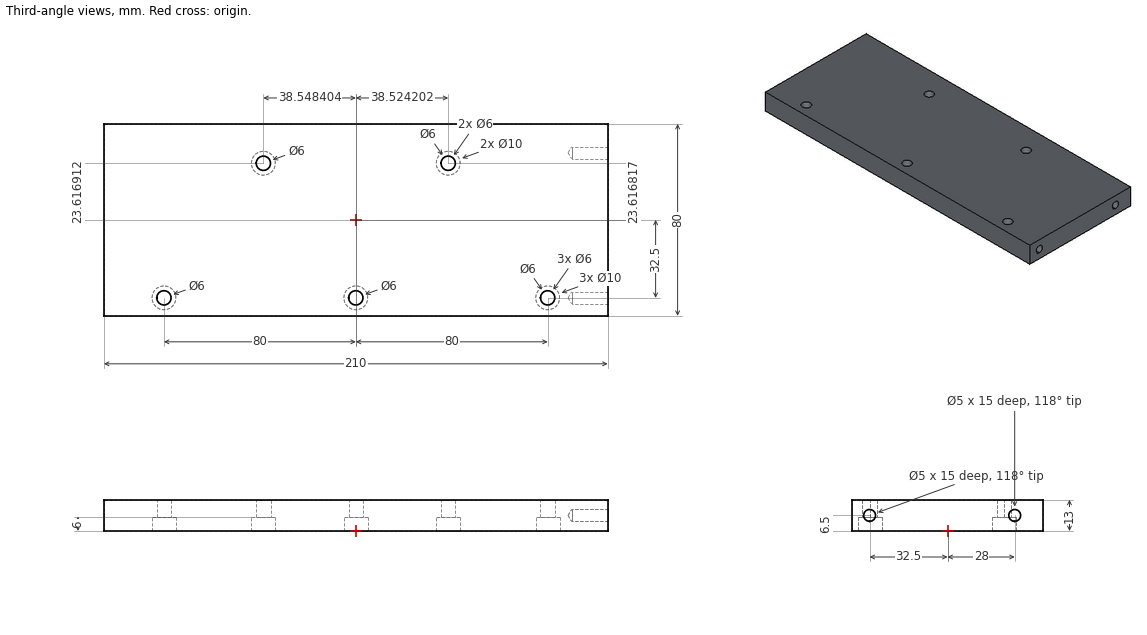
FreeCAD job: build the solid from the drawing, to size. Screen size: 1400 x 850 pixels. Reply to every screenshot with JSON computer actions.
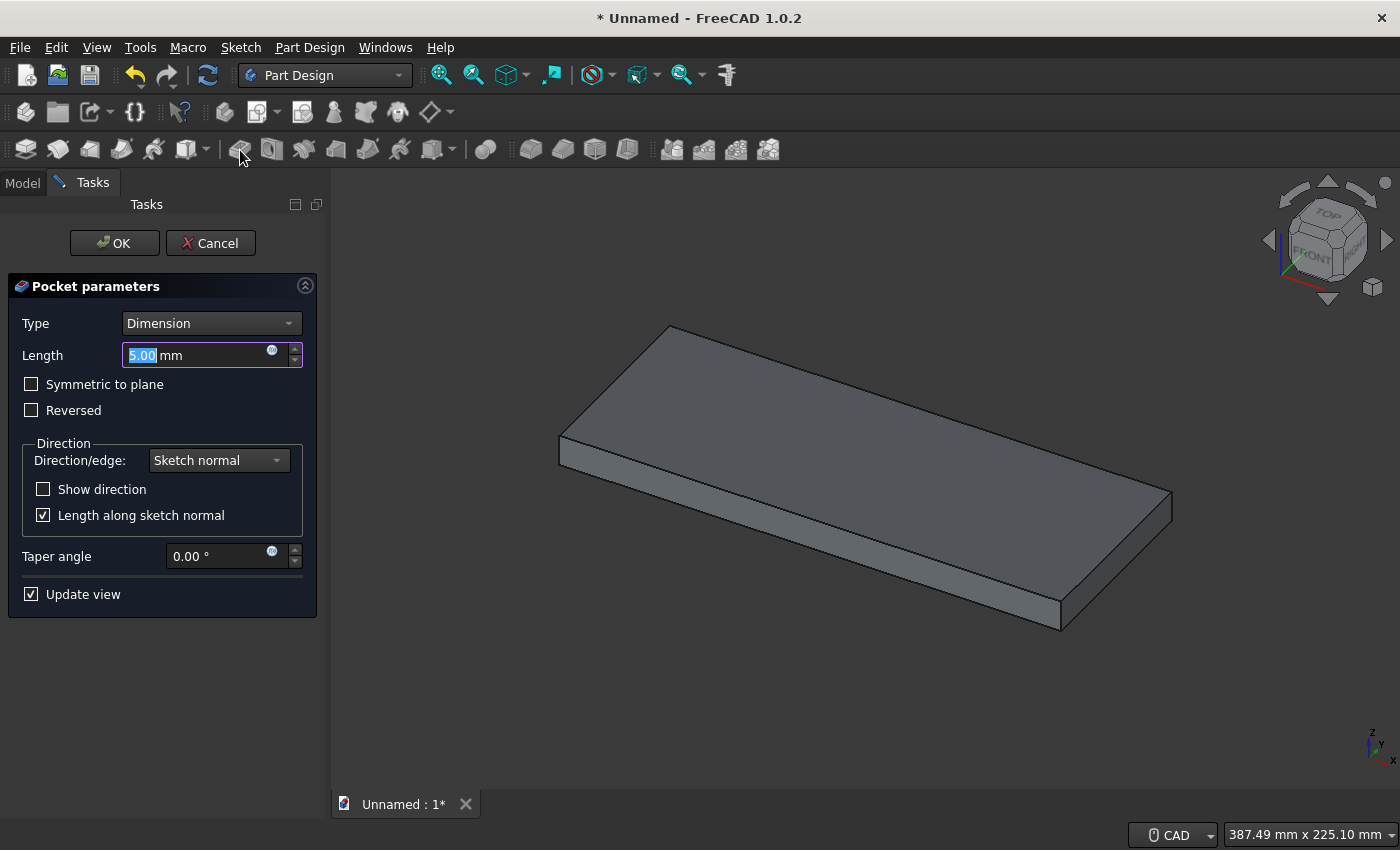
{"action": "type", "text": "6"}
{"action": "key", "text": "Tab"}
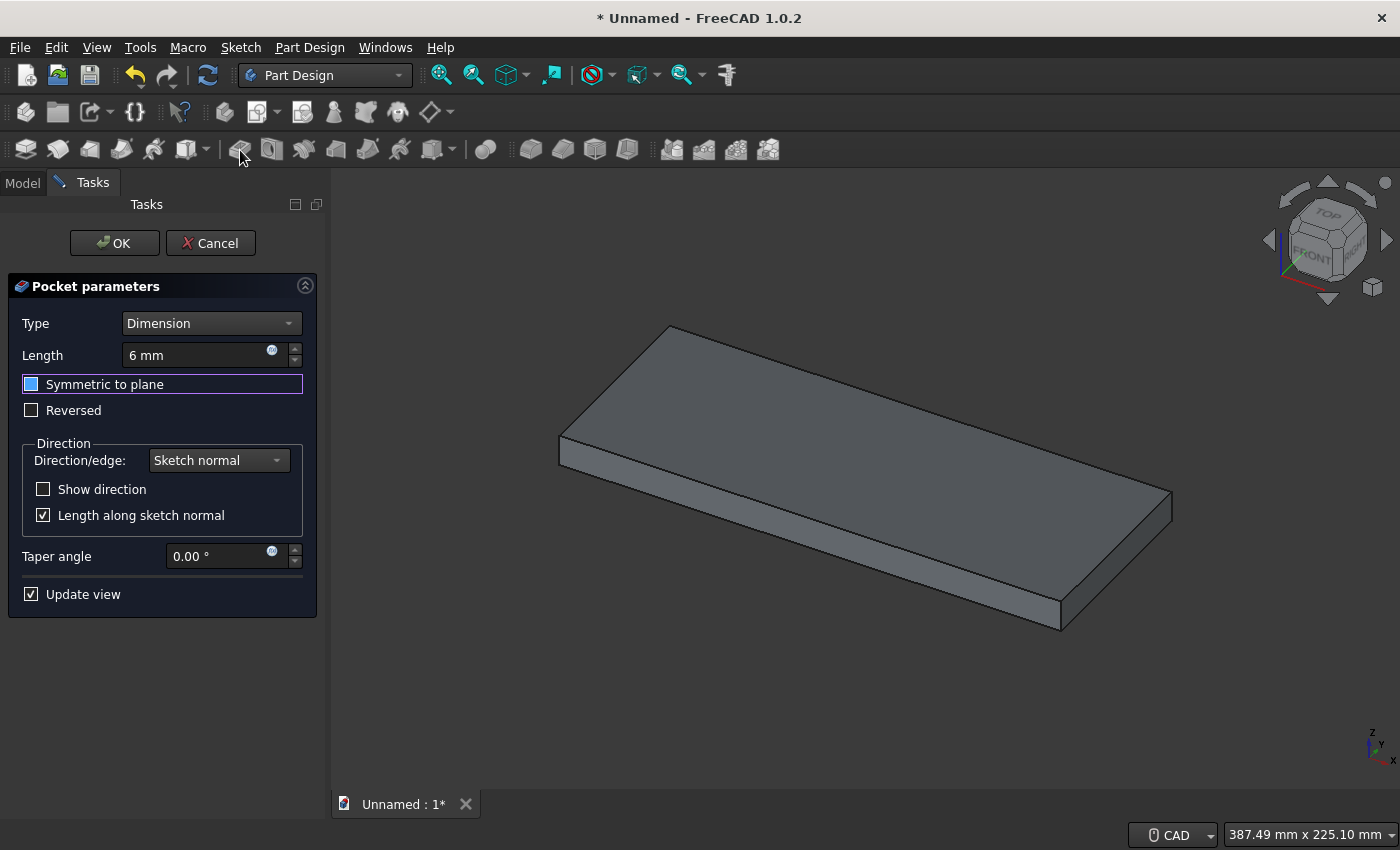
{"action": "left_click", "coordinate": [30, 410]}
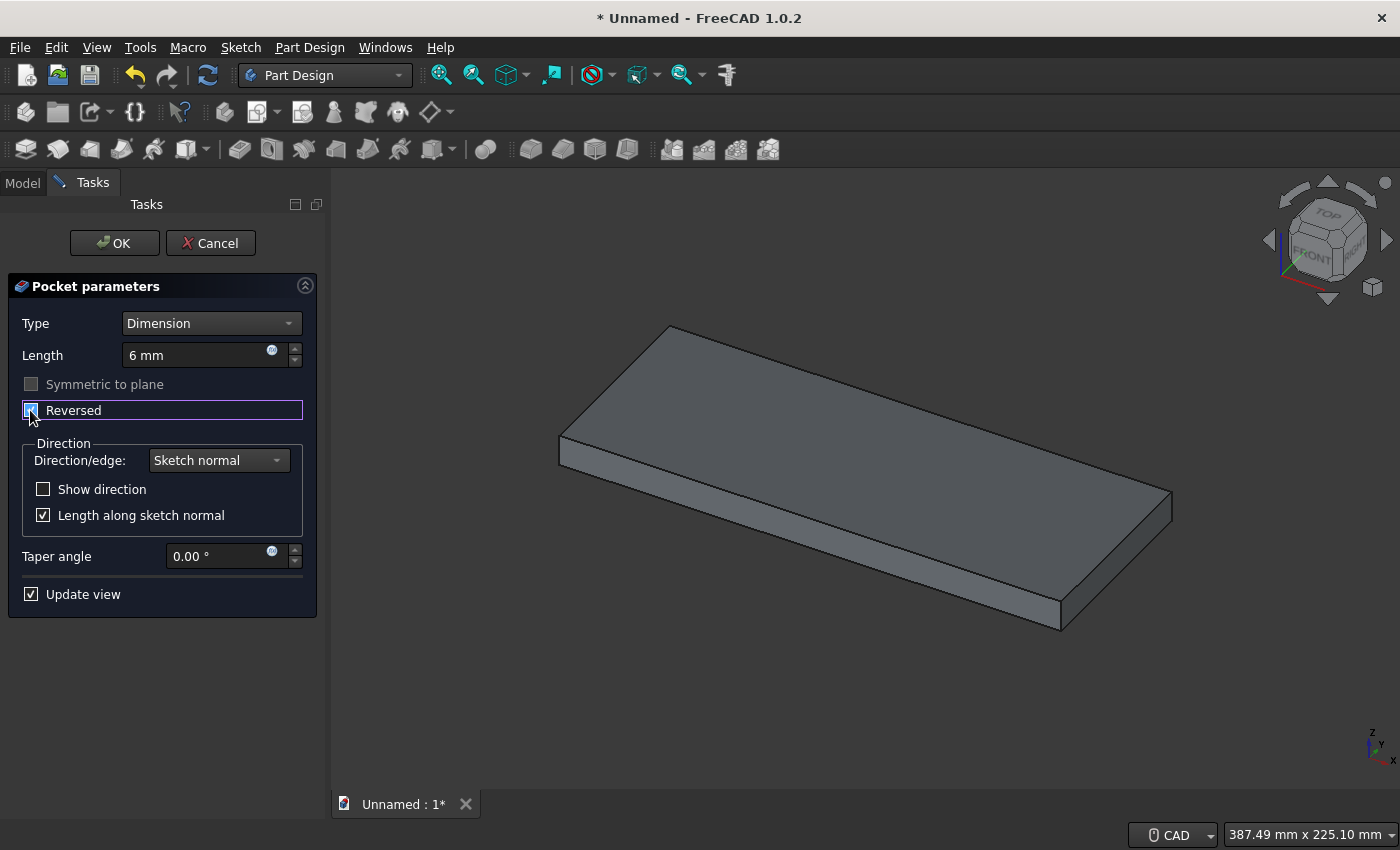
{"action": "left_click", "coordinate": [115, 243]}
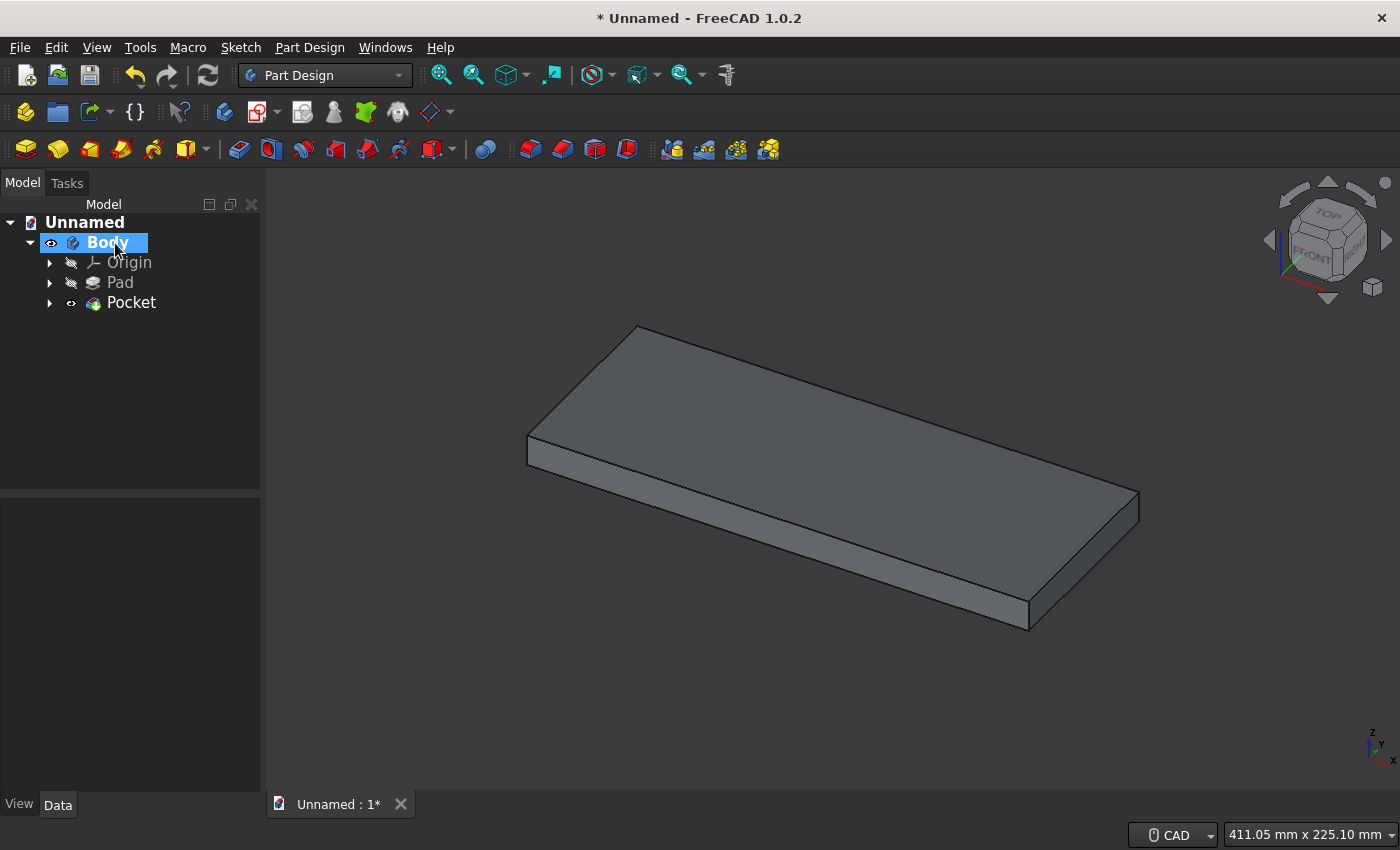
{"action": "left_click", "coordinate": [258, 112]}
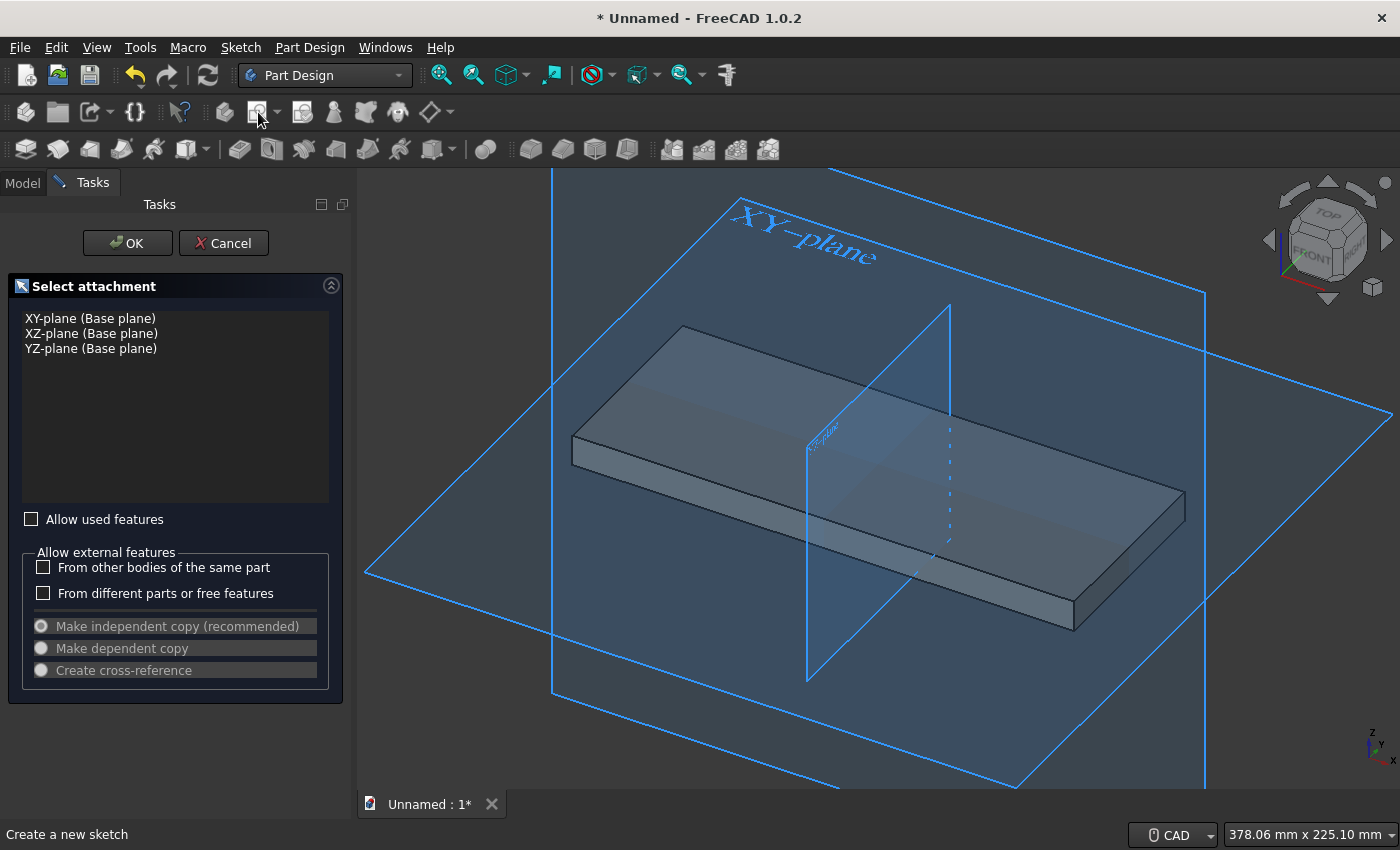
{"action": "left_click", "coordinate": [82, 318]}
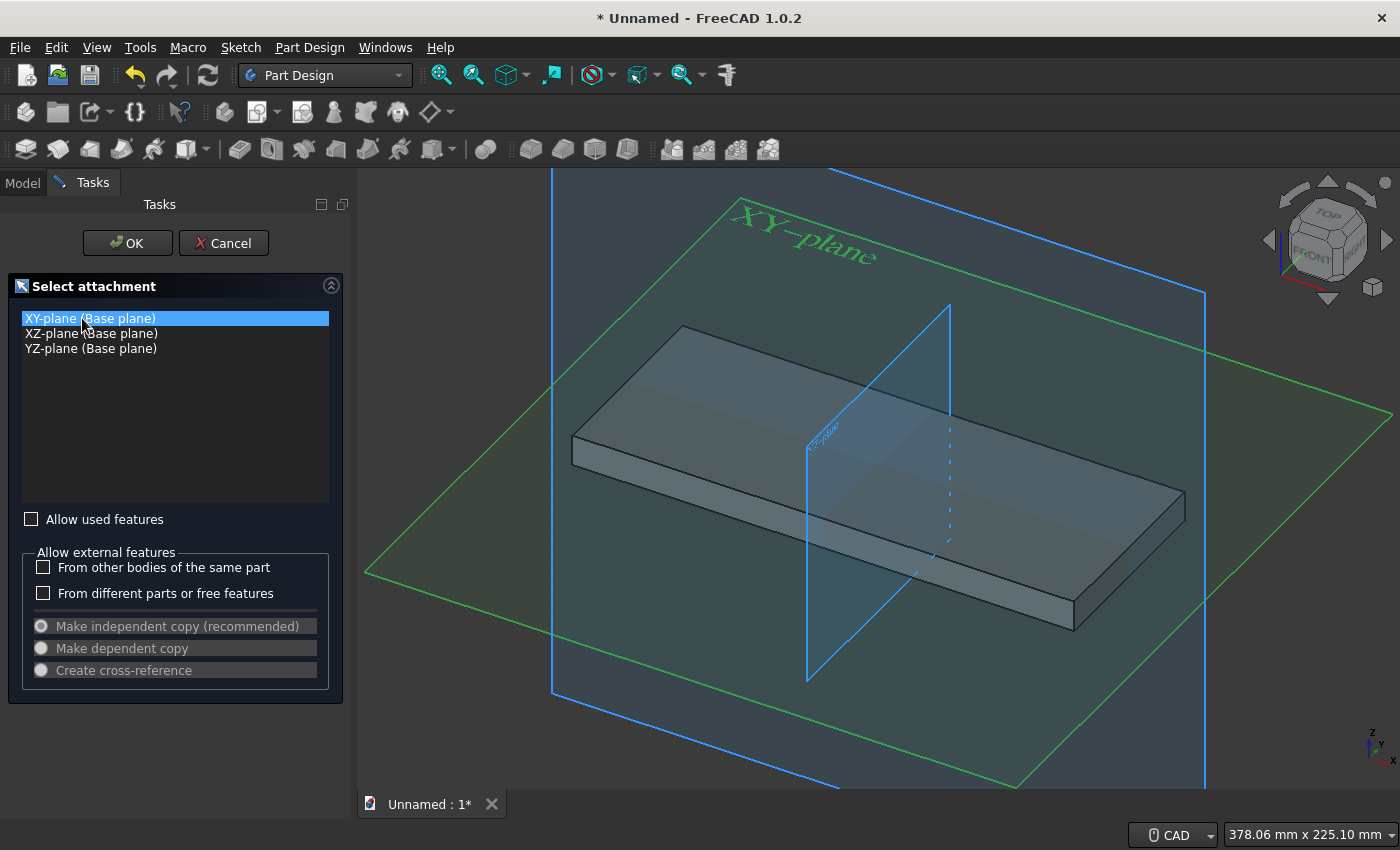
{"action": "left_click", "coordinate": [128, 243]}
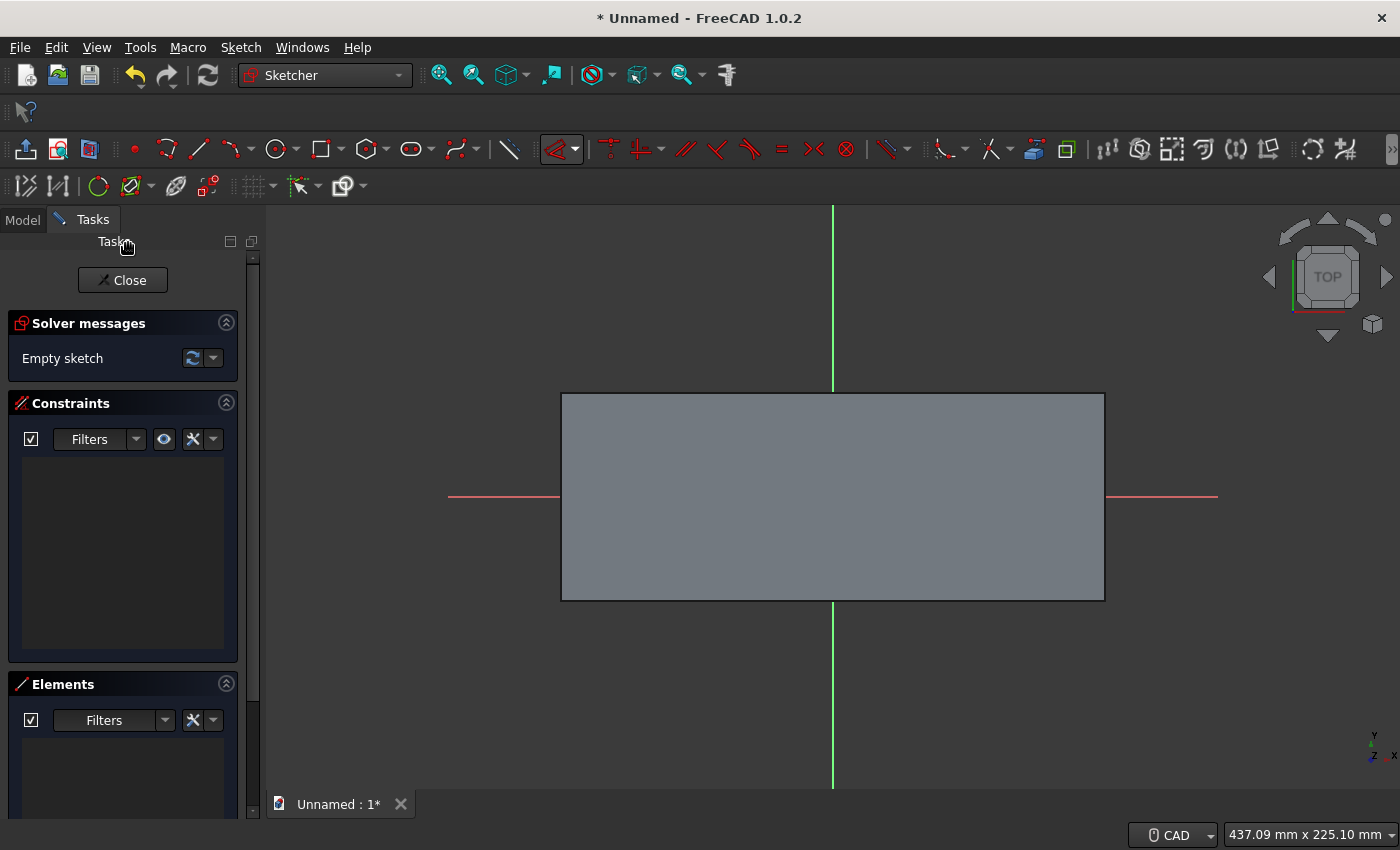
{"action": "left_click", "coordinate": [90, 150]}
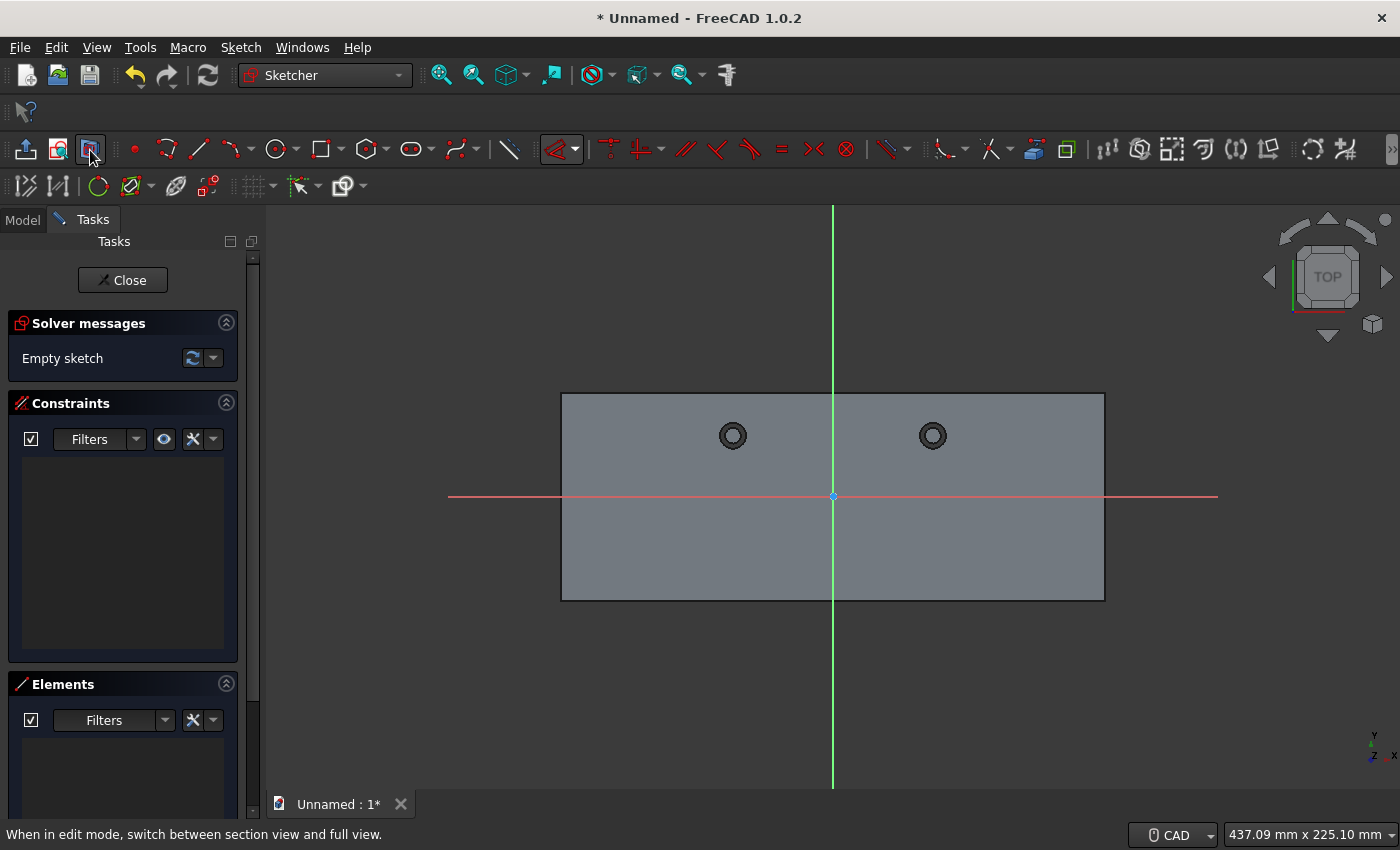
{"action": "scroll", "coordinate": [942, 433], "scroll_direction": "up", "scroll_amount": 15}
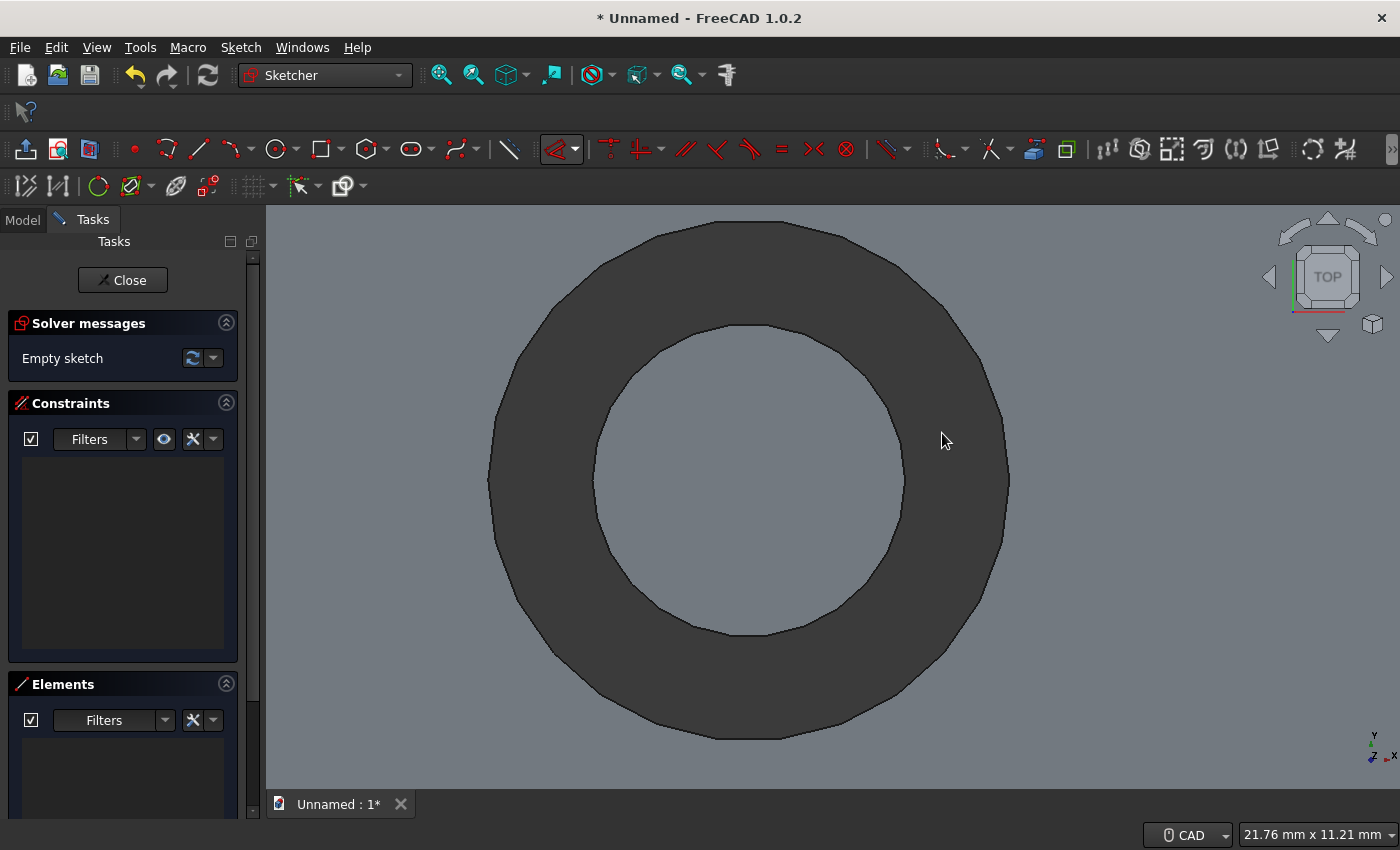
{"action": "key", "text": "g c"}